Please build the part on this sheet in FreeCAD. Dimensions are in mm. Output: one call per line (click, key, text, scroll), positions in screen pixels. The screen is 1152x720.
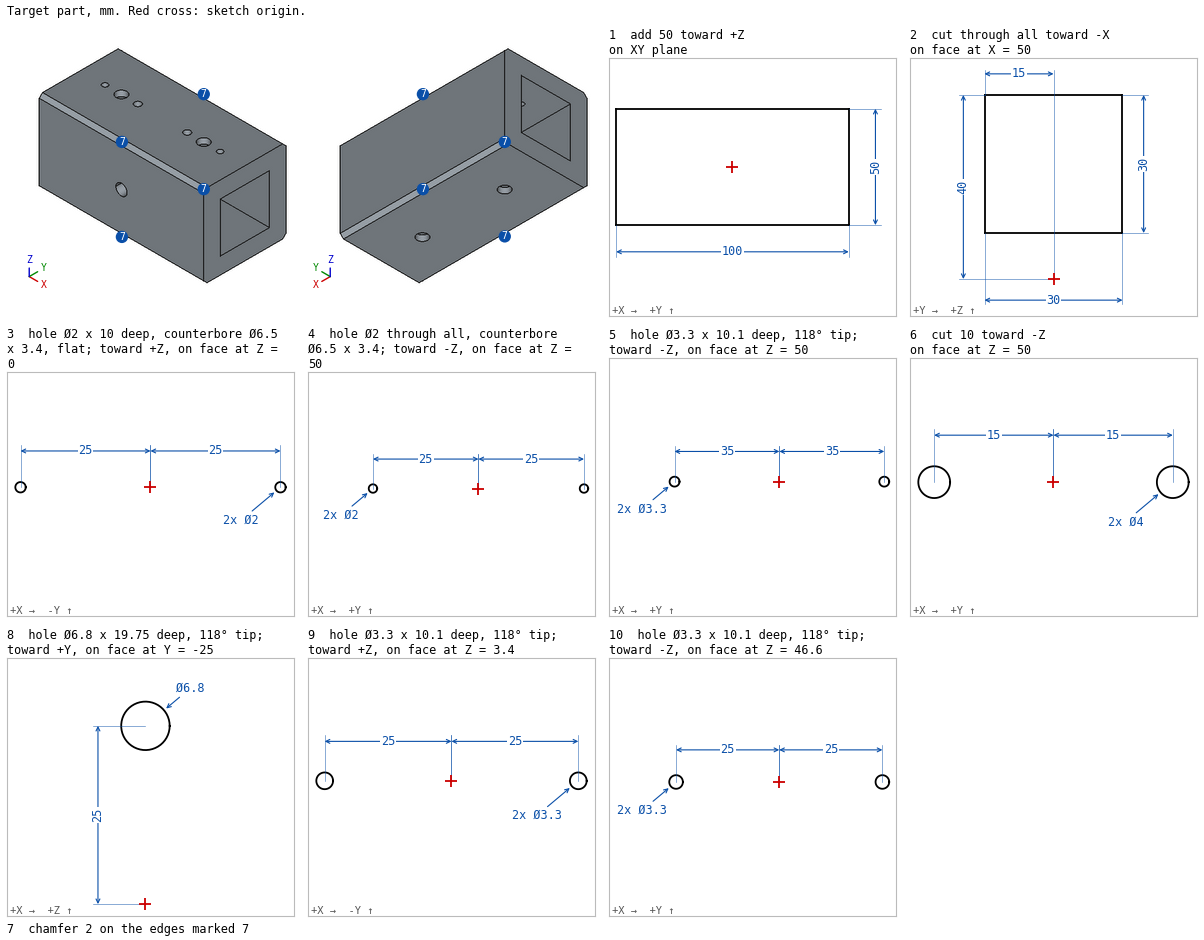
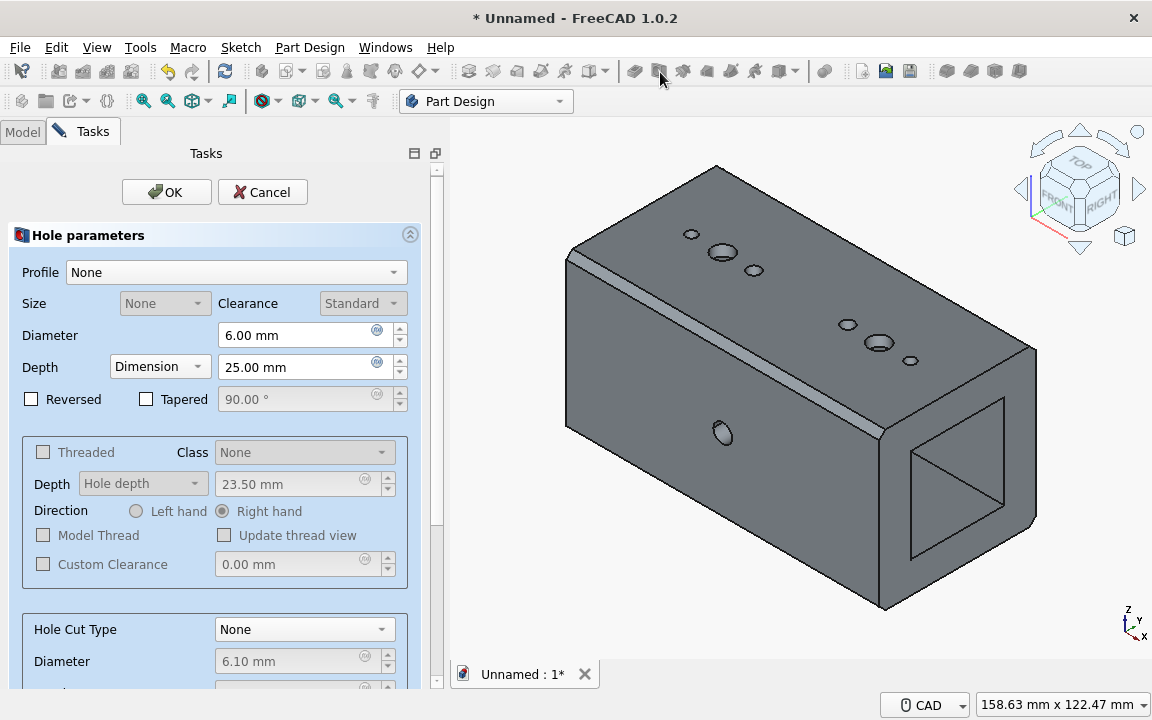
triple_click(305, 335)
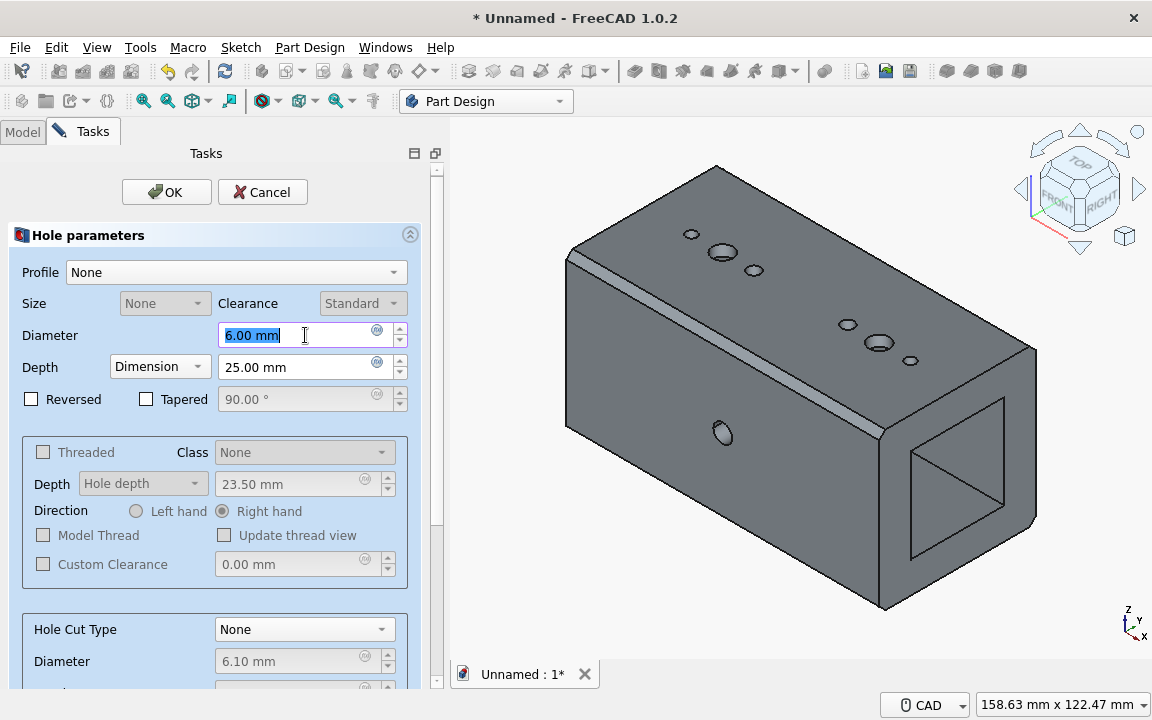
text(6.8)
key(Tab)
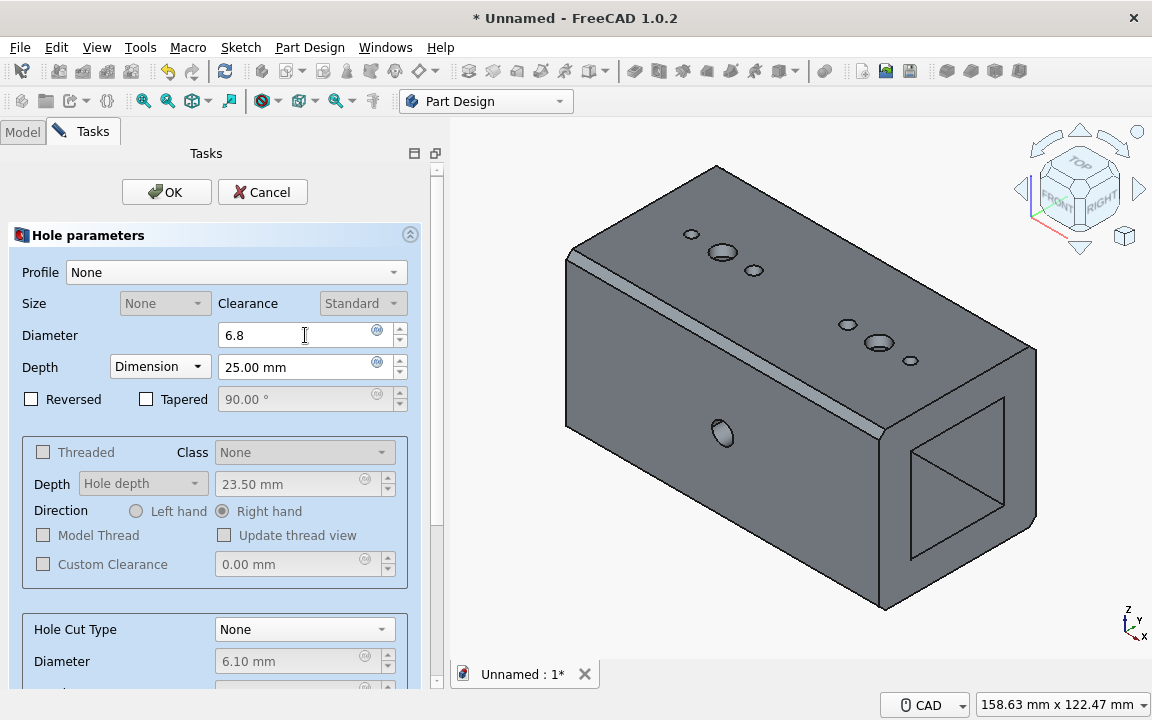
triple_click(305, 367)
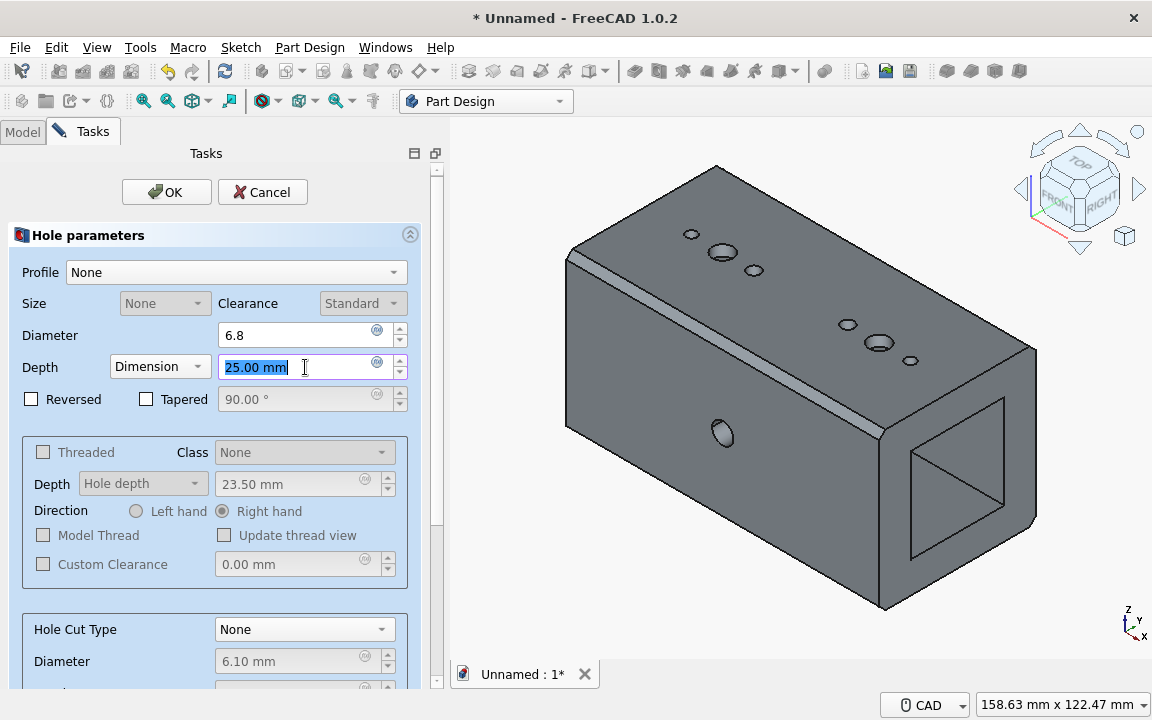
text(19.75)
key(Tab)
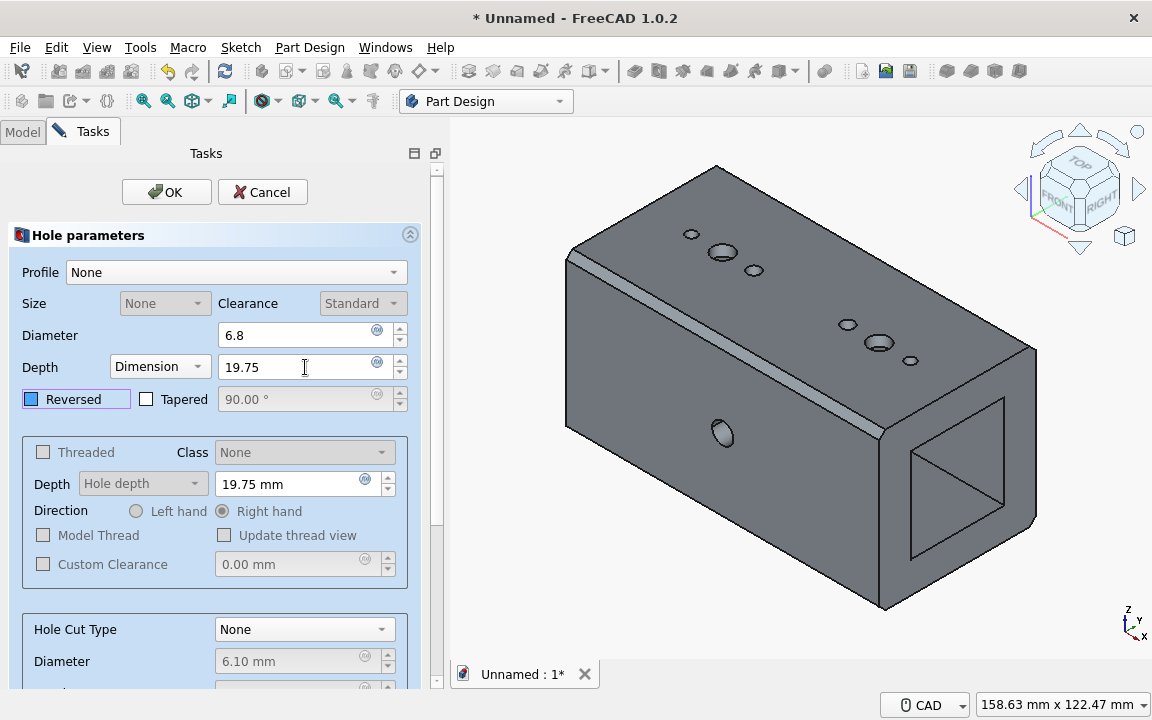
click(167, 192)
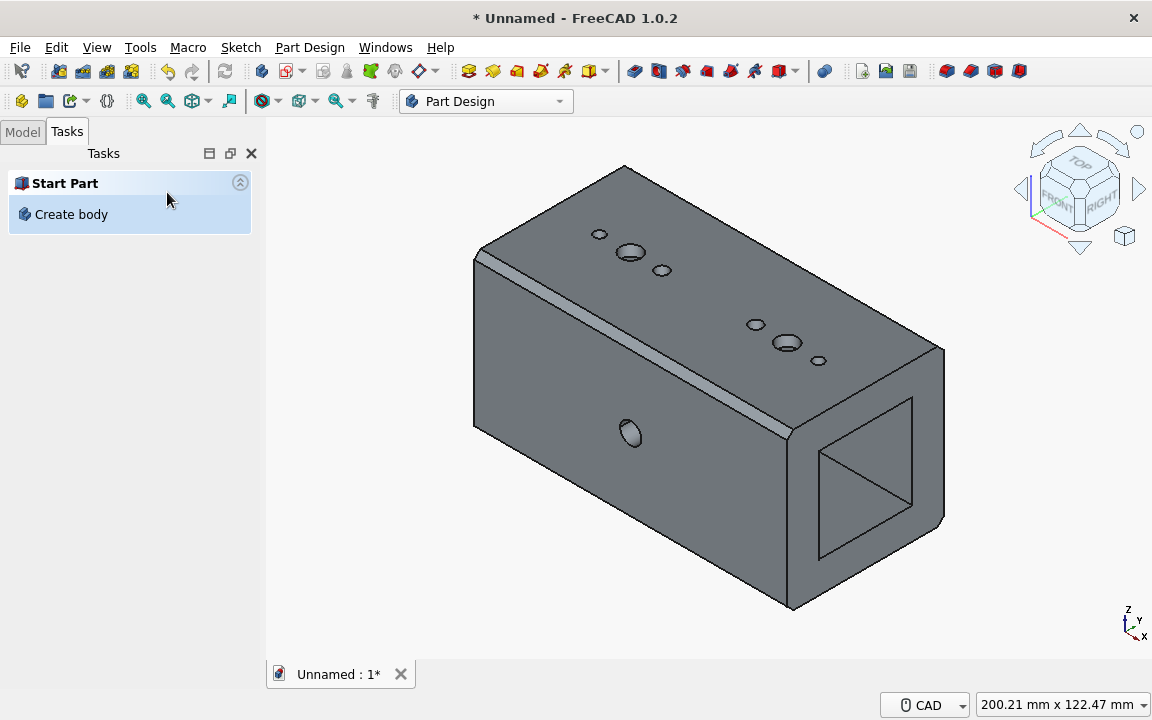
key(5)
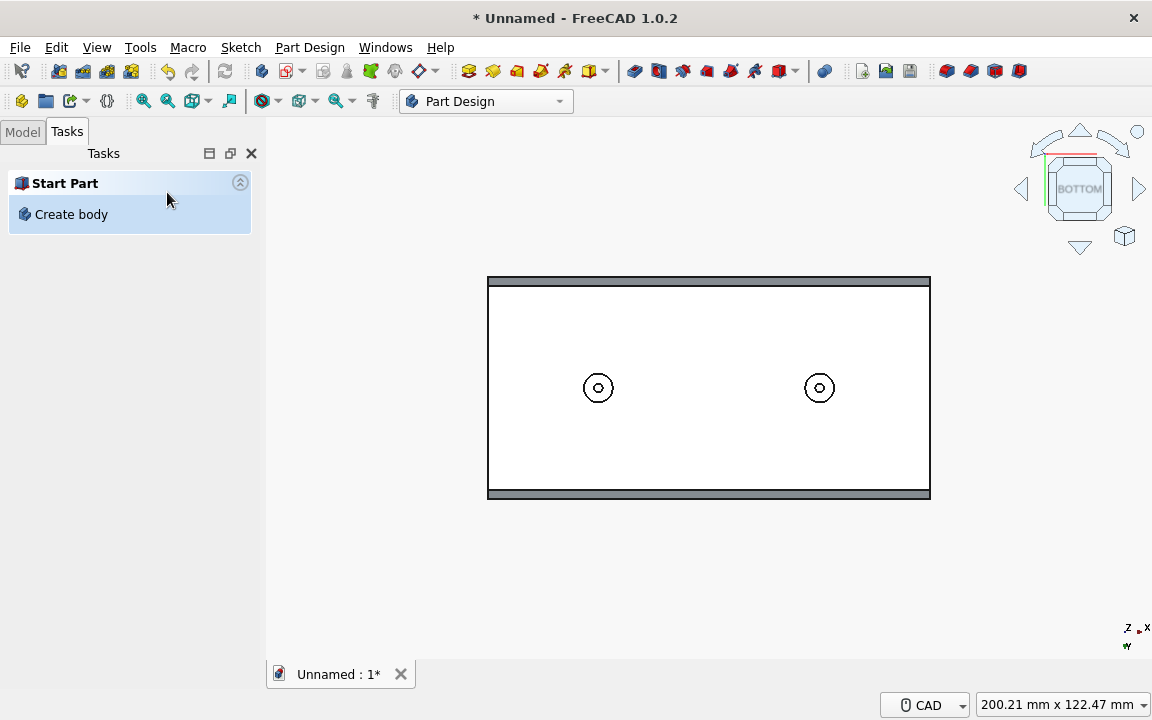
scroll(816, 379, up, 5)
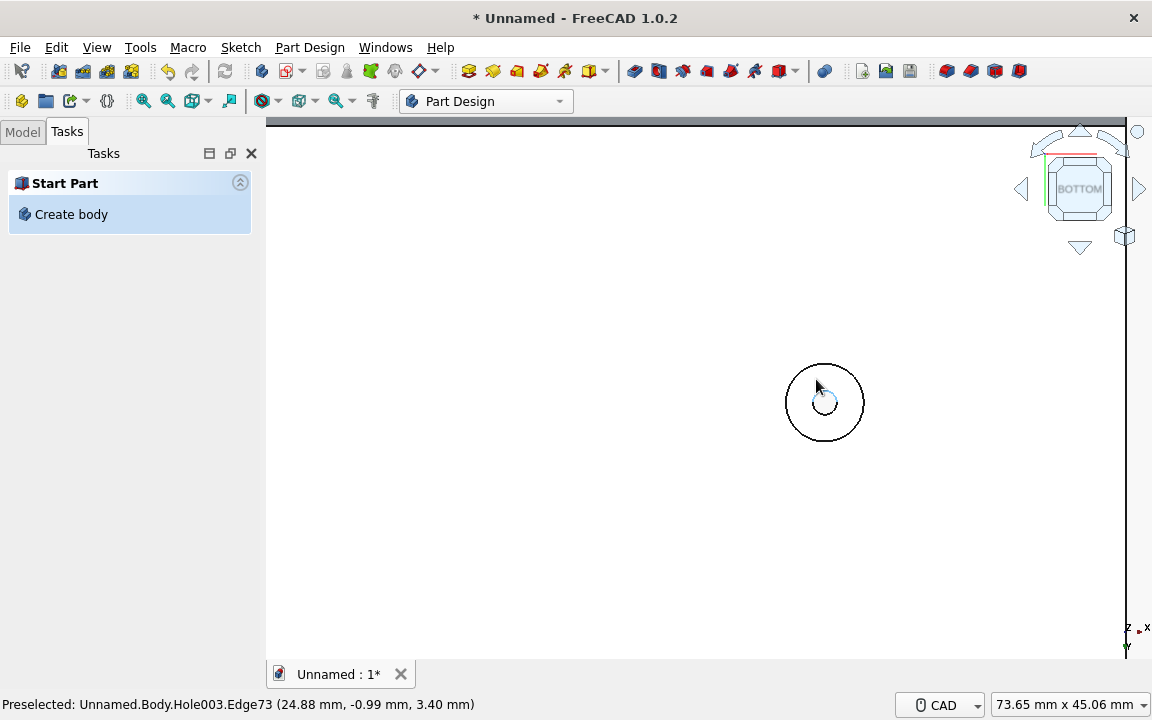
click(814, 379)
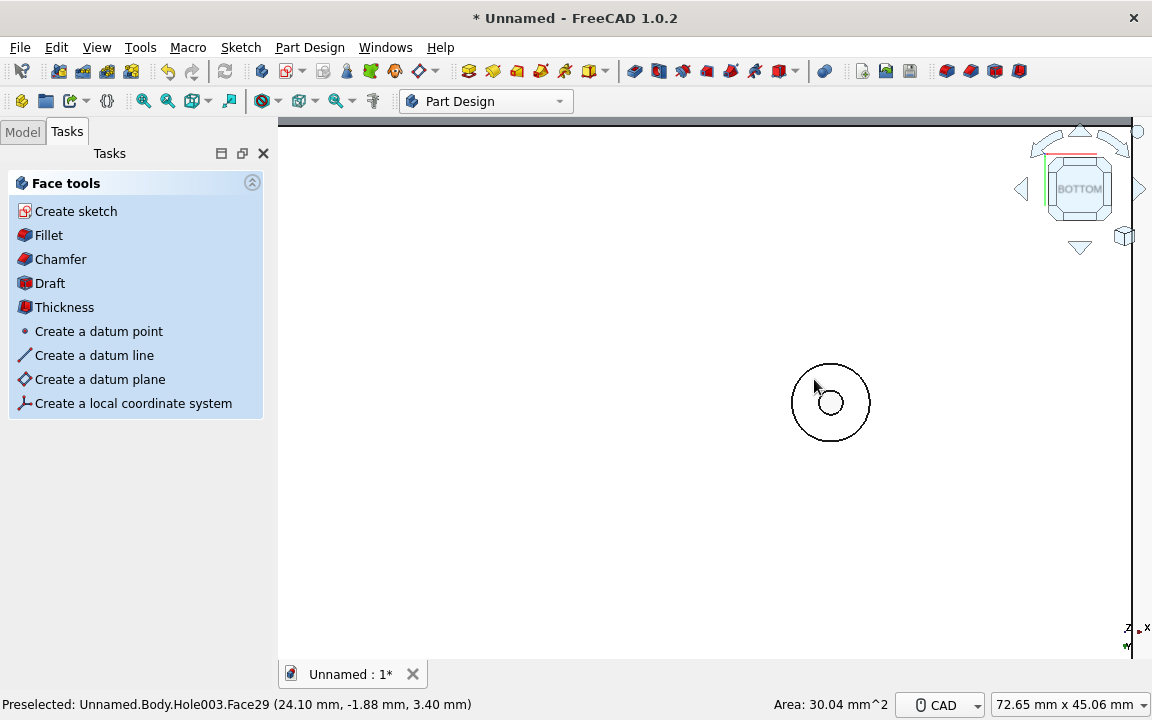
click(286, 72)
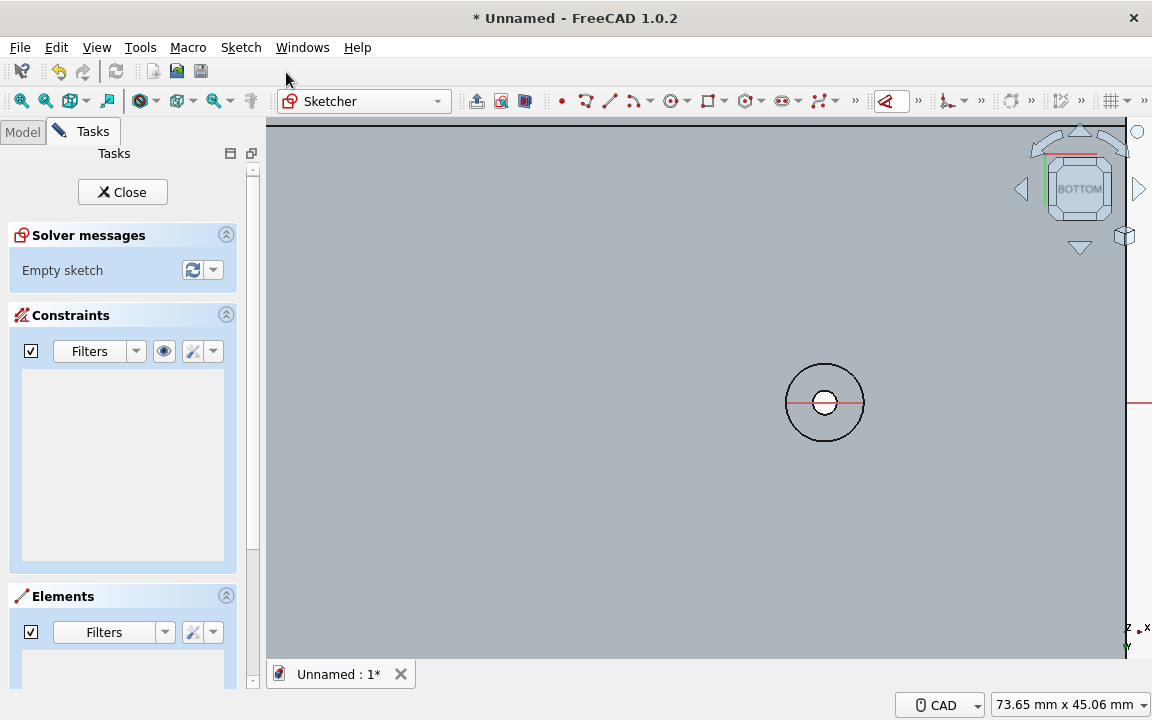
click(526, 102)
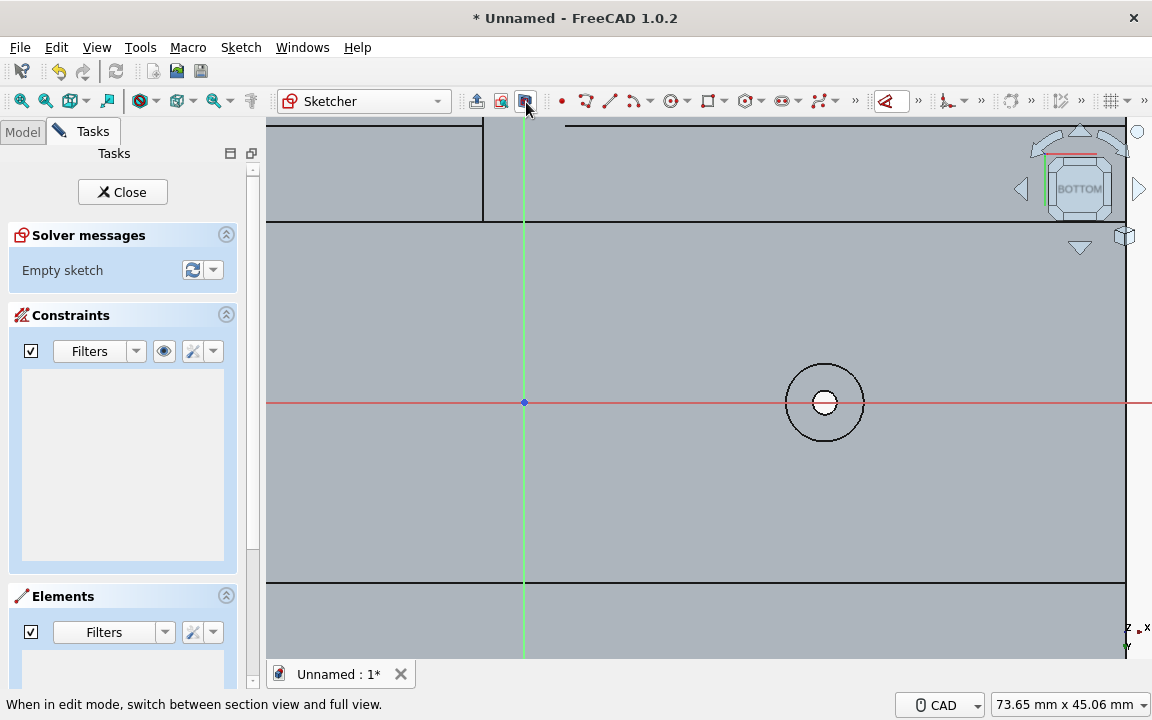
scroll(987, 322, down, 1)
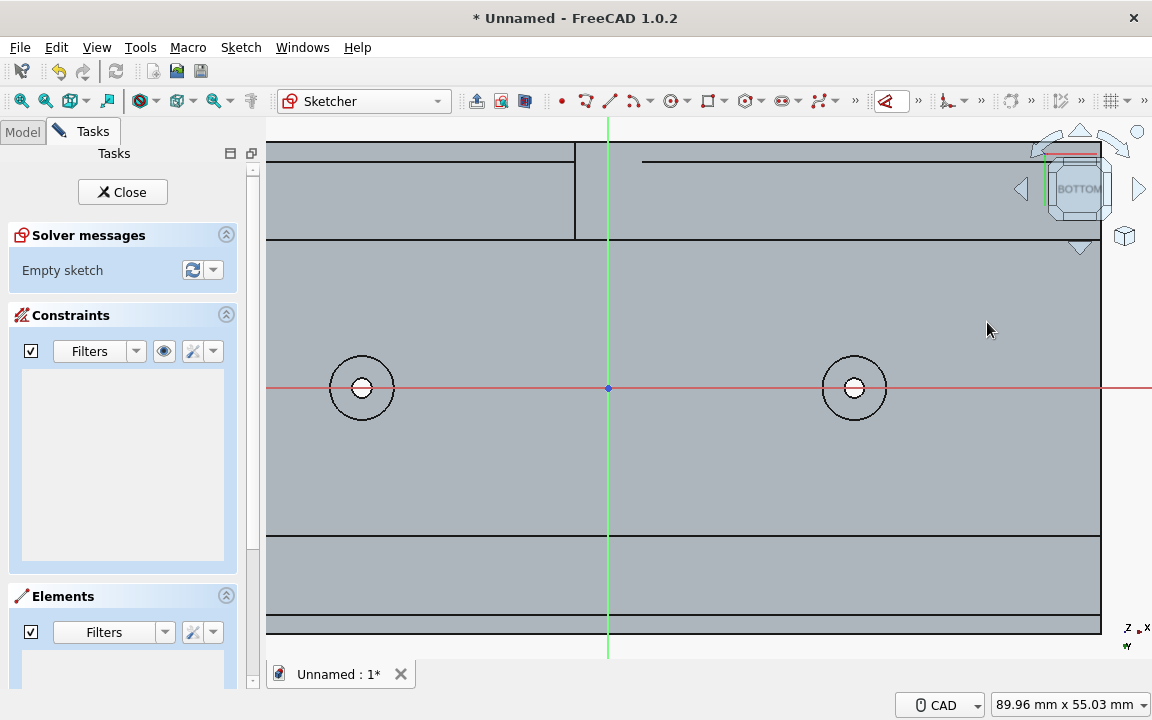
click(672, 102)